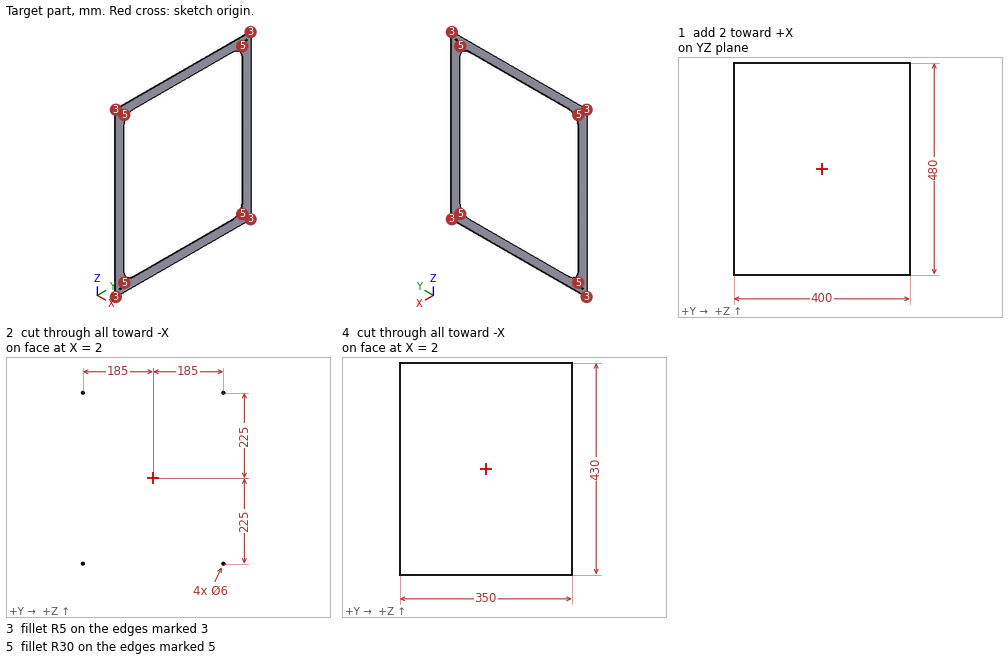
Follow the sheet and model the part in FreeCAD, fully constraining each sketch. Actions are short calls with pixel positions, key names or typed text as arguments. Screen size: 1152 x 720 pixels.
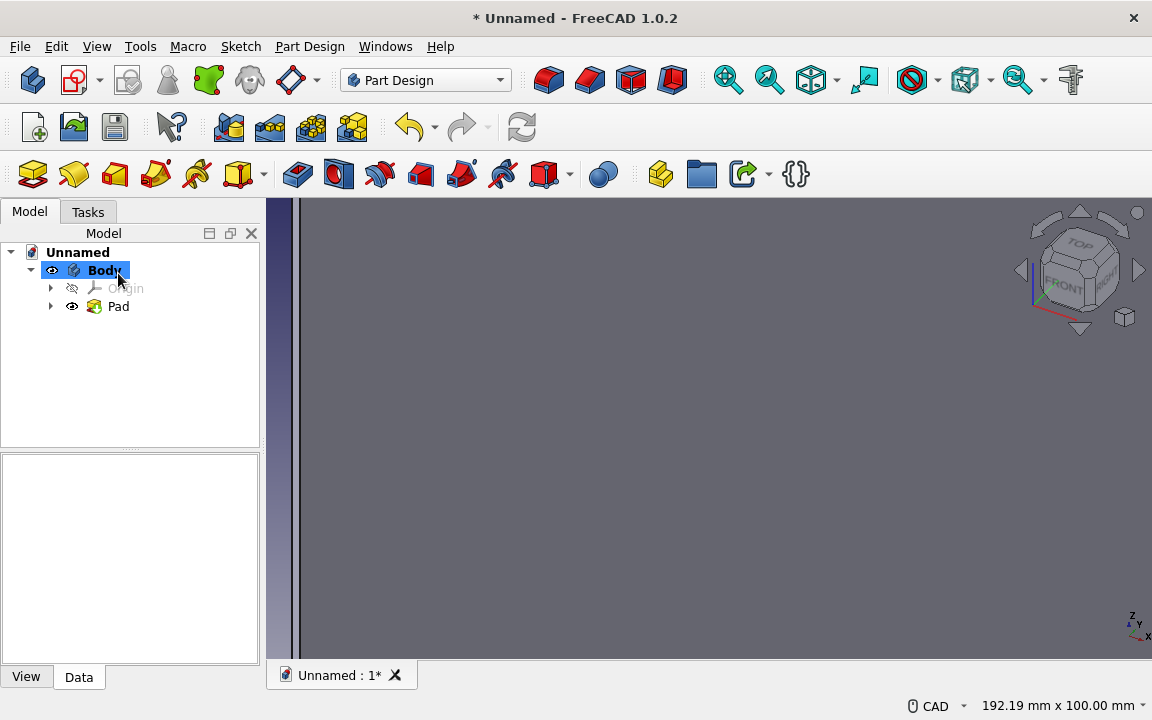
click(729, 80)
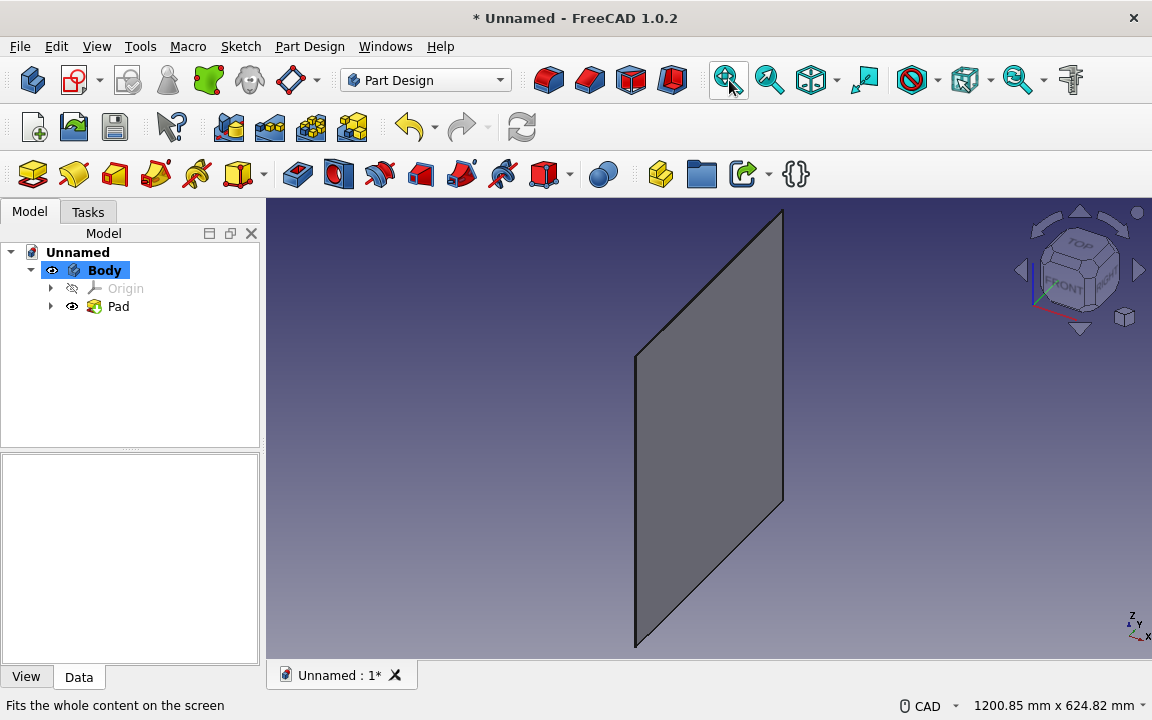
click(710, 428)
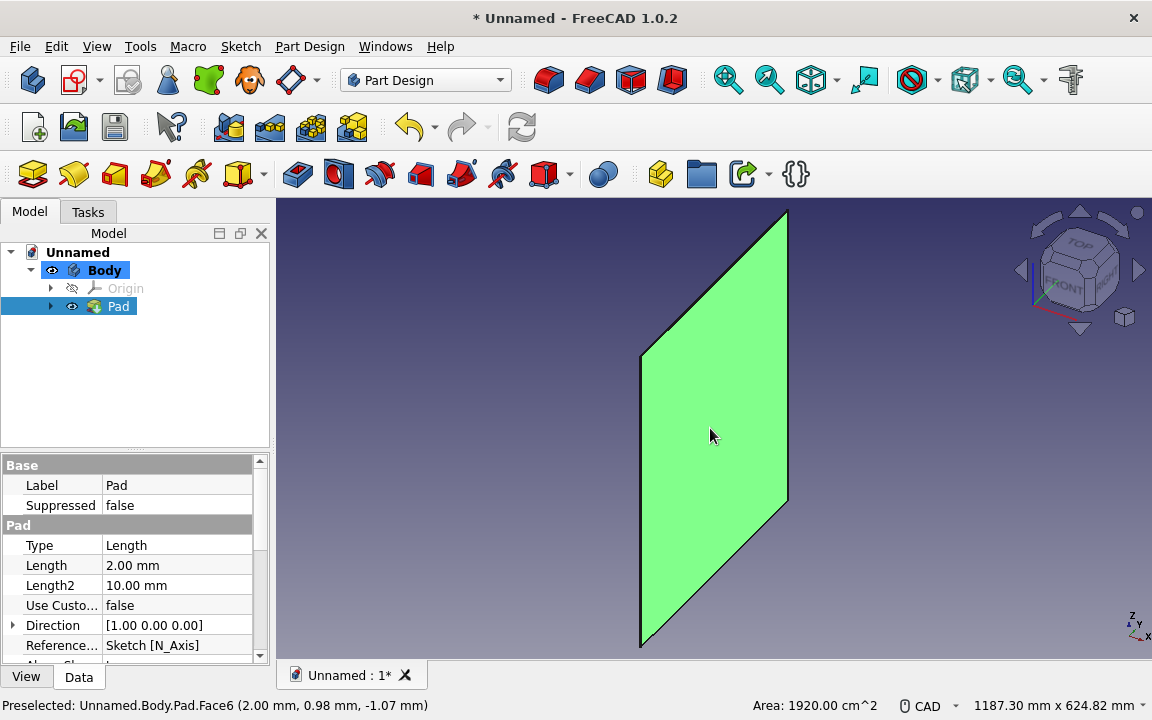
click(74, 80)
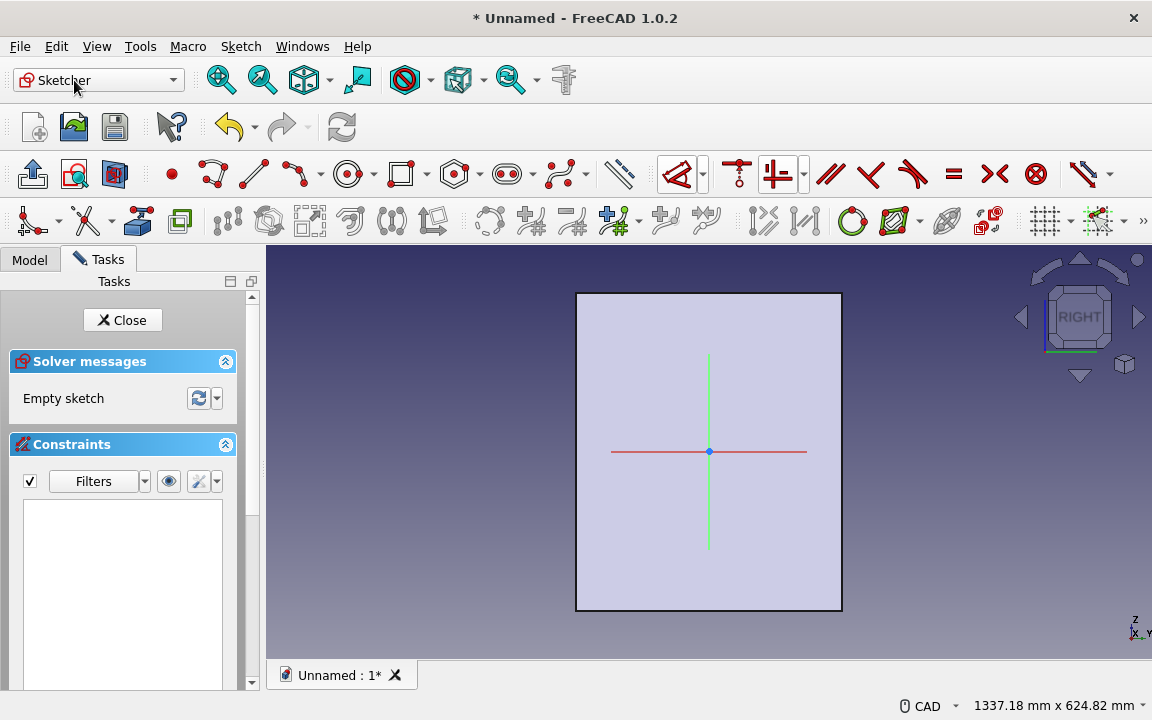
click(348, 174)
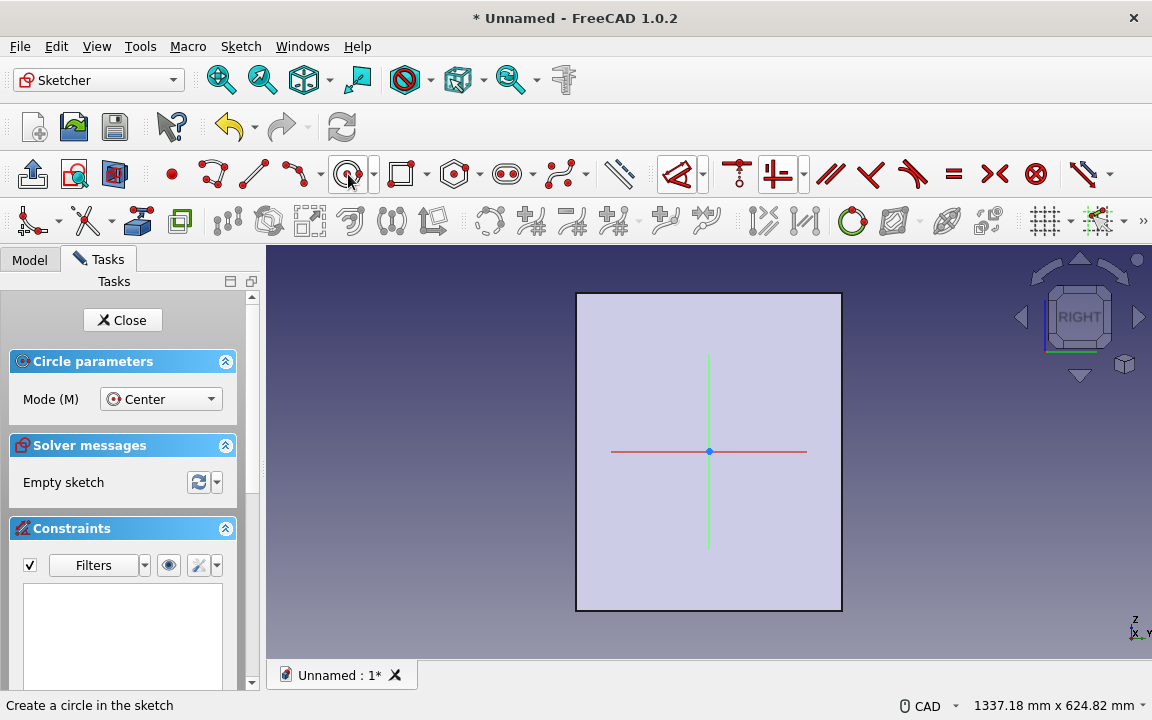
scroll(832, 303, up, 13)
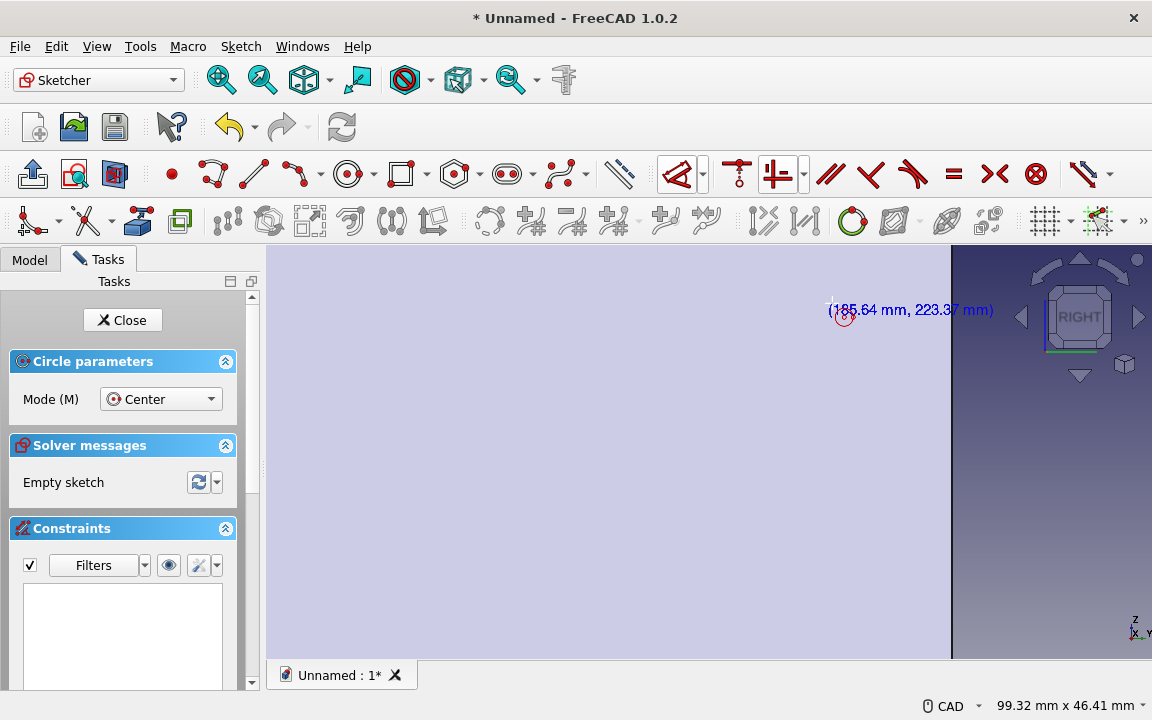
scroll(736, 332, down, 14)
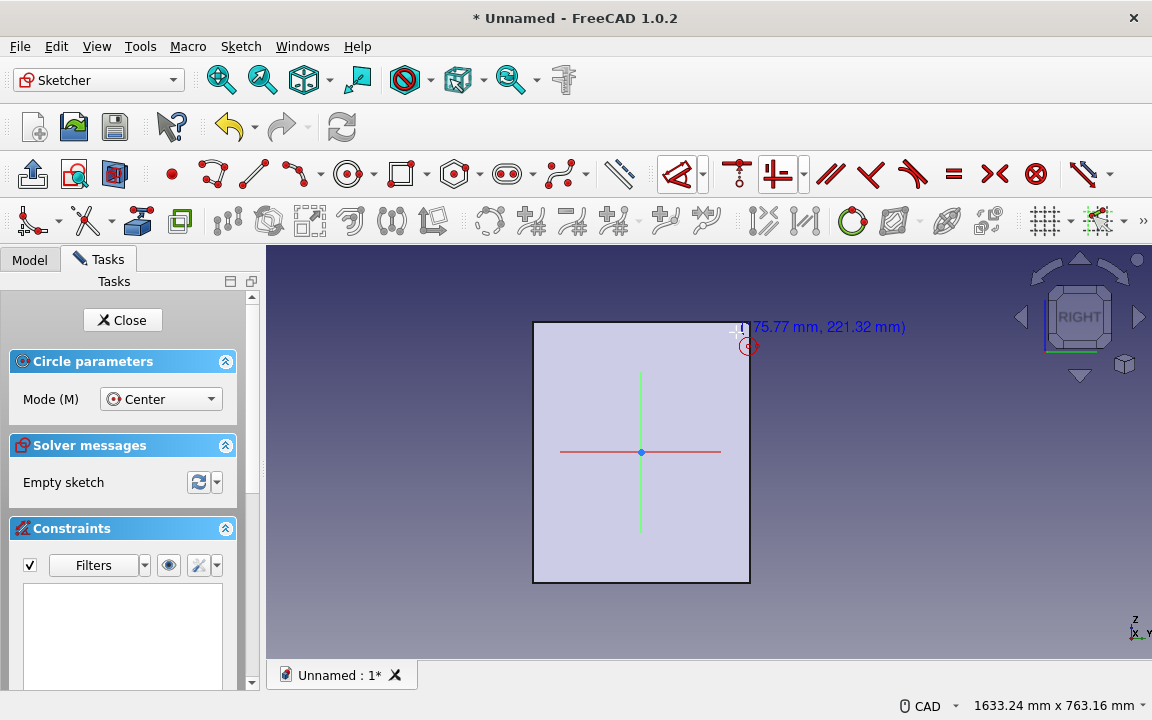
click(742, 330)
move(743, 329)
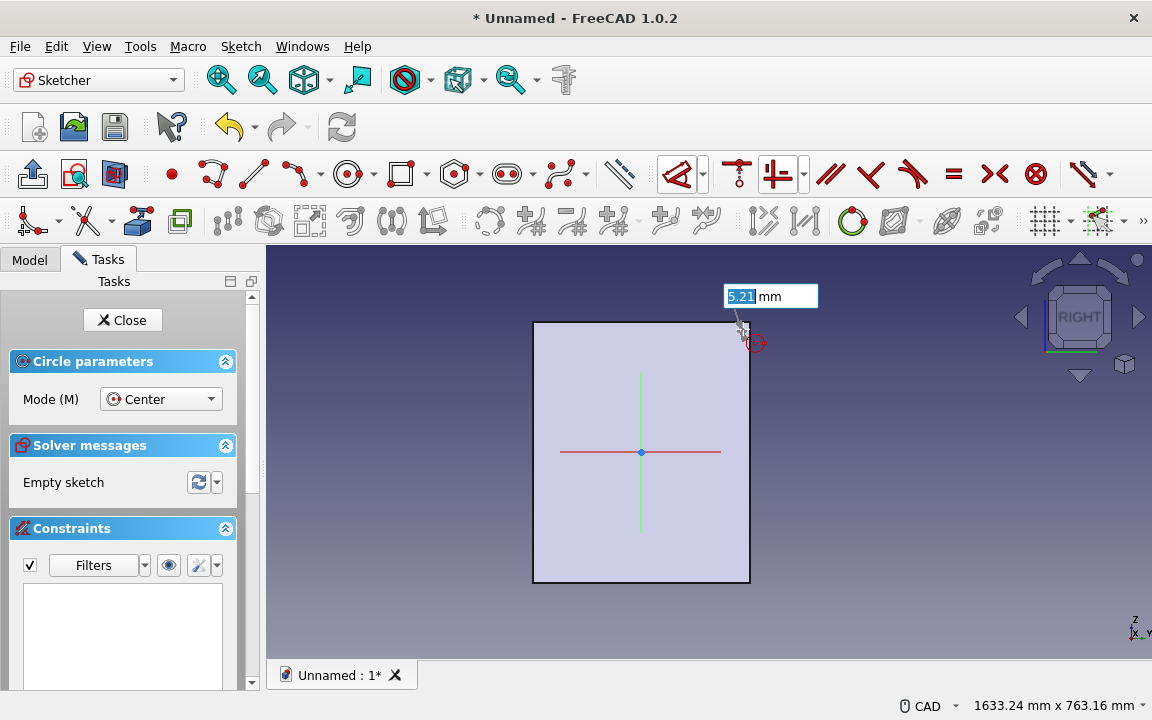
text(6)
key(Return)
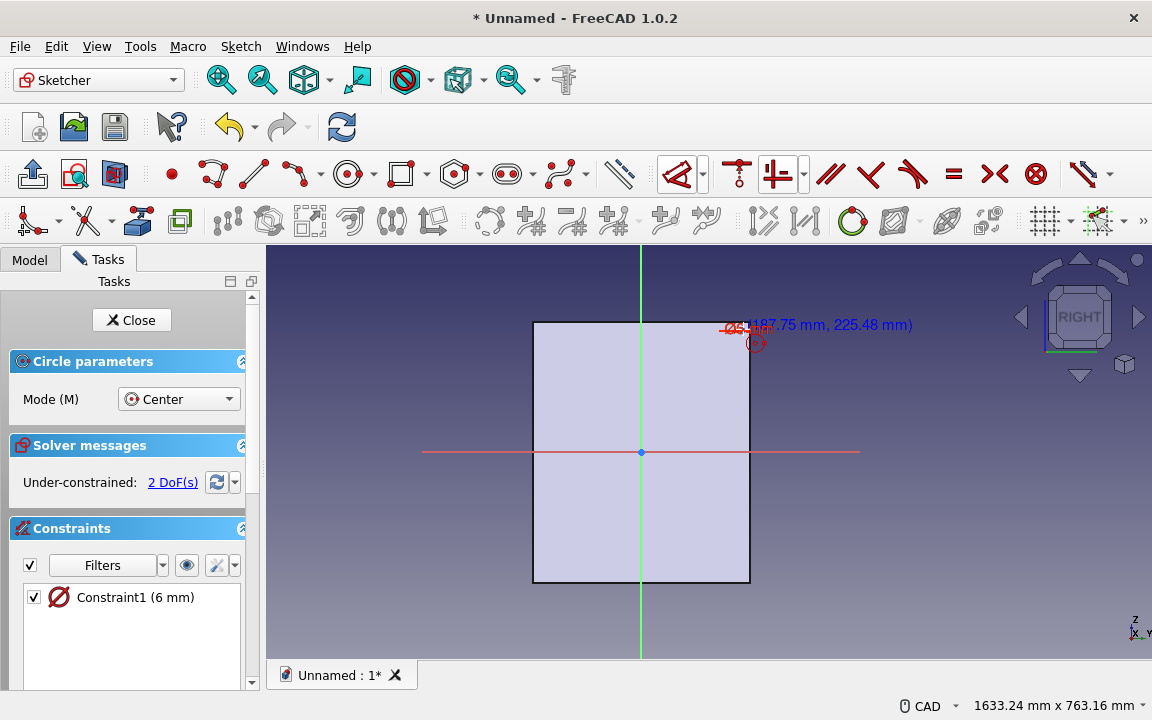
scroll(742, 574, up, 14)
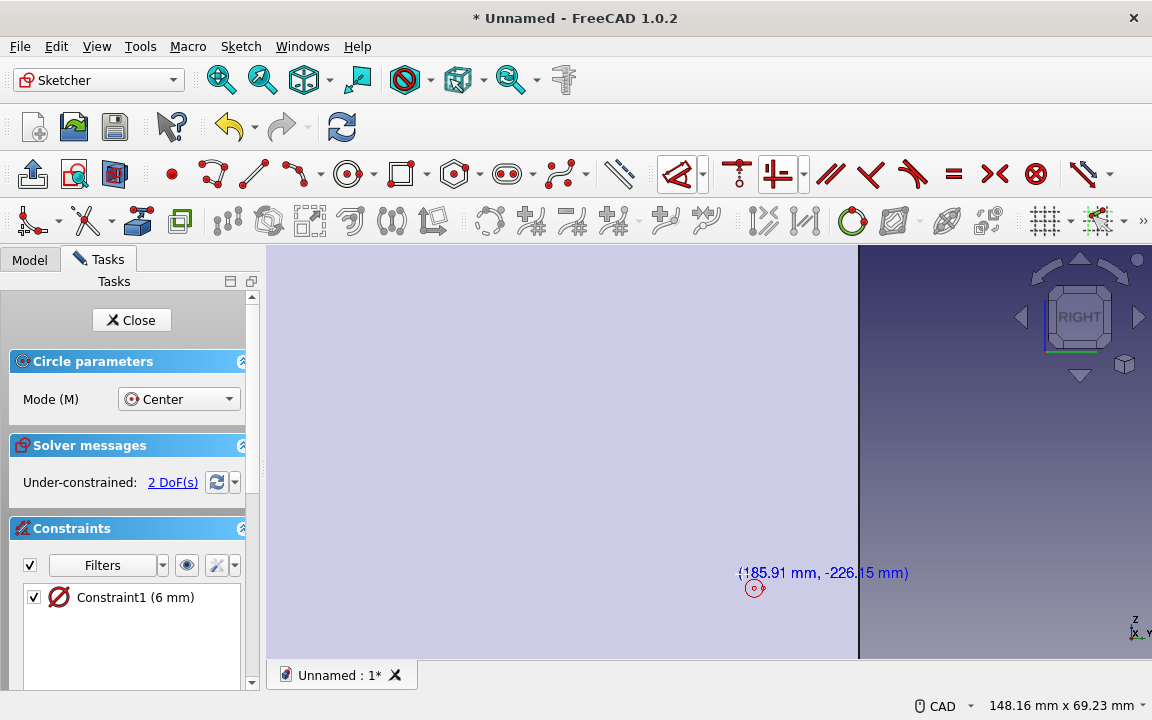
scroll(742, 574, down, 14)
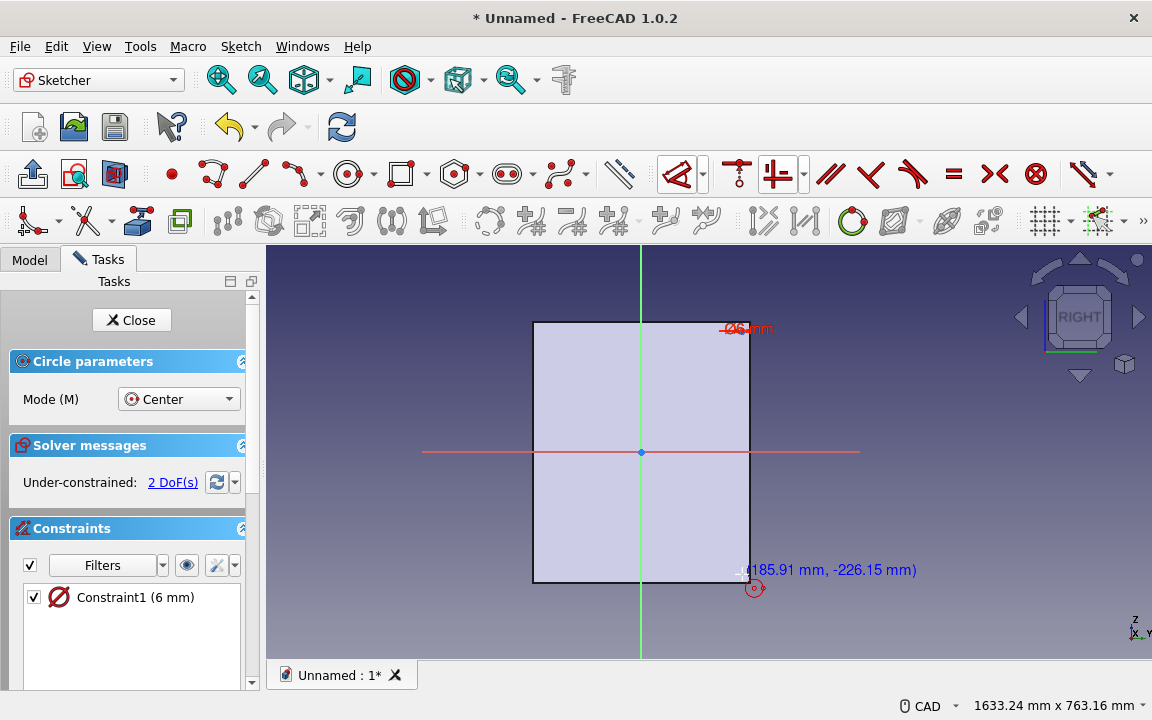
click(742, 574)
move(743, 573)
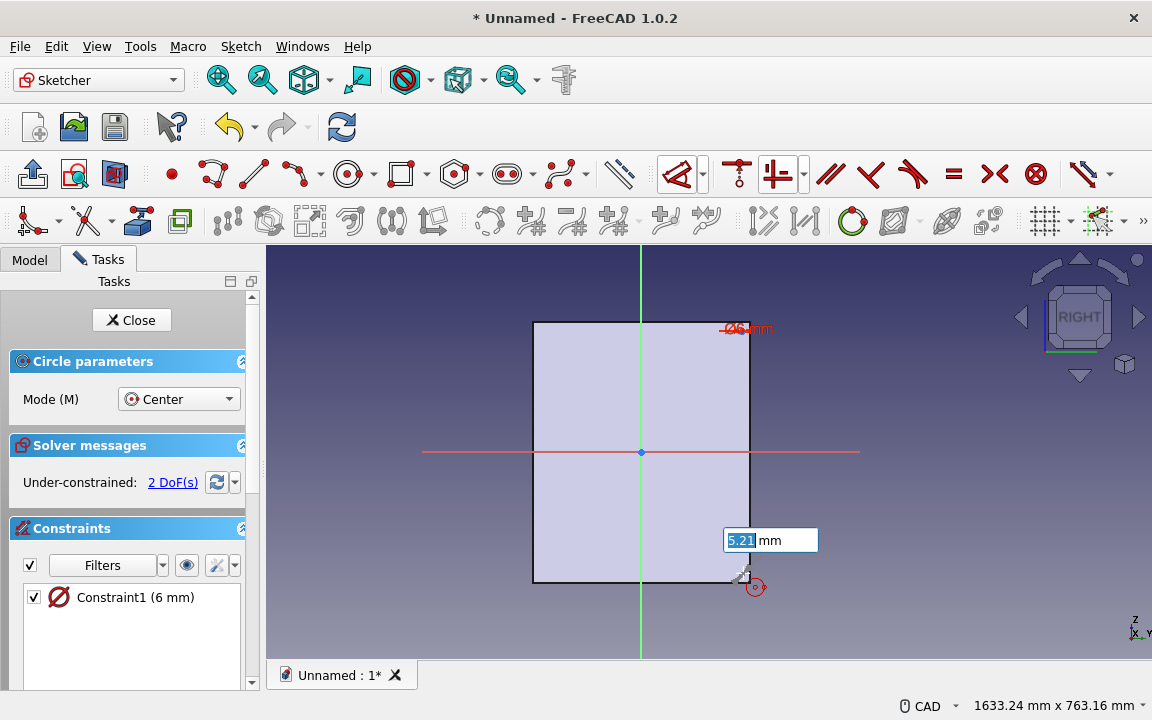
text(6)
key(Return)